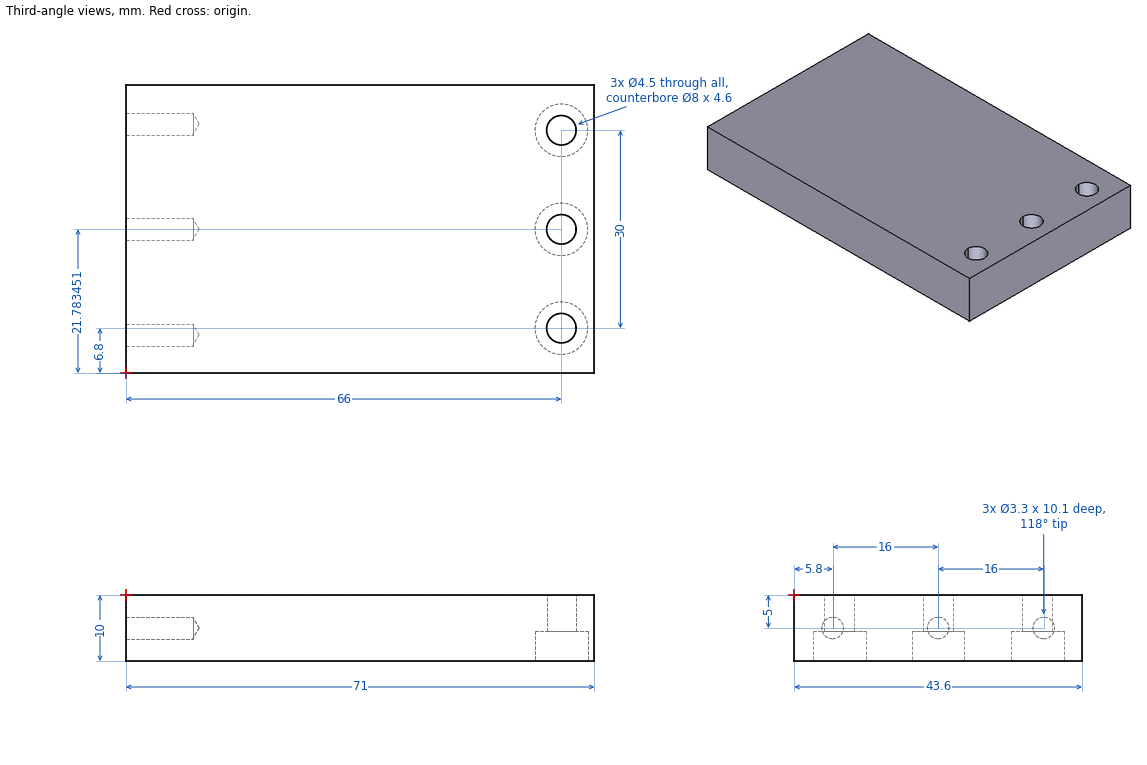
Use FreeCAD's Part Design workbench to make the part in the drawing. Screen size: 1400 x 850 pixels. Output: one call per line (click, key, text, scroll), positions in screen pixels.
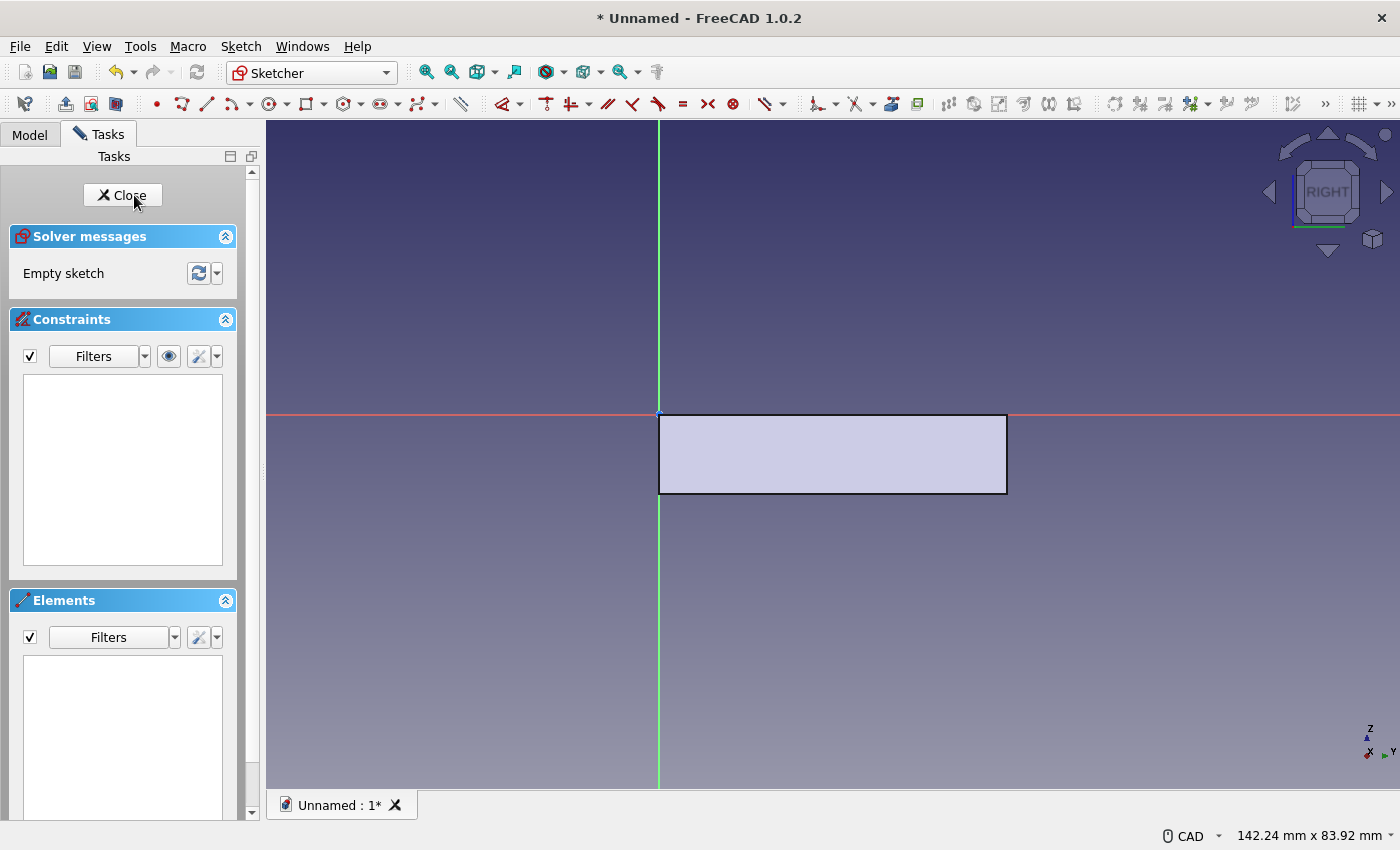
key(q)
key(s)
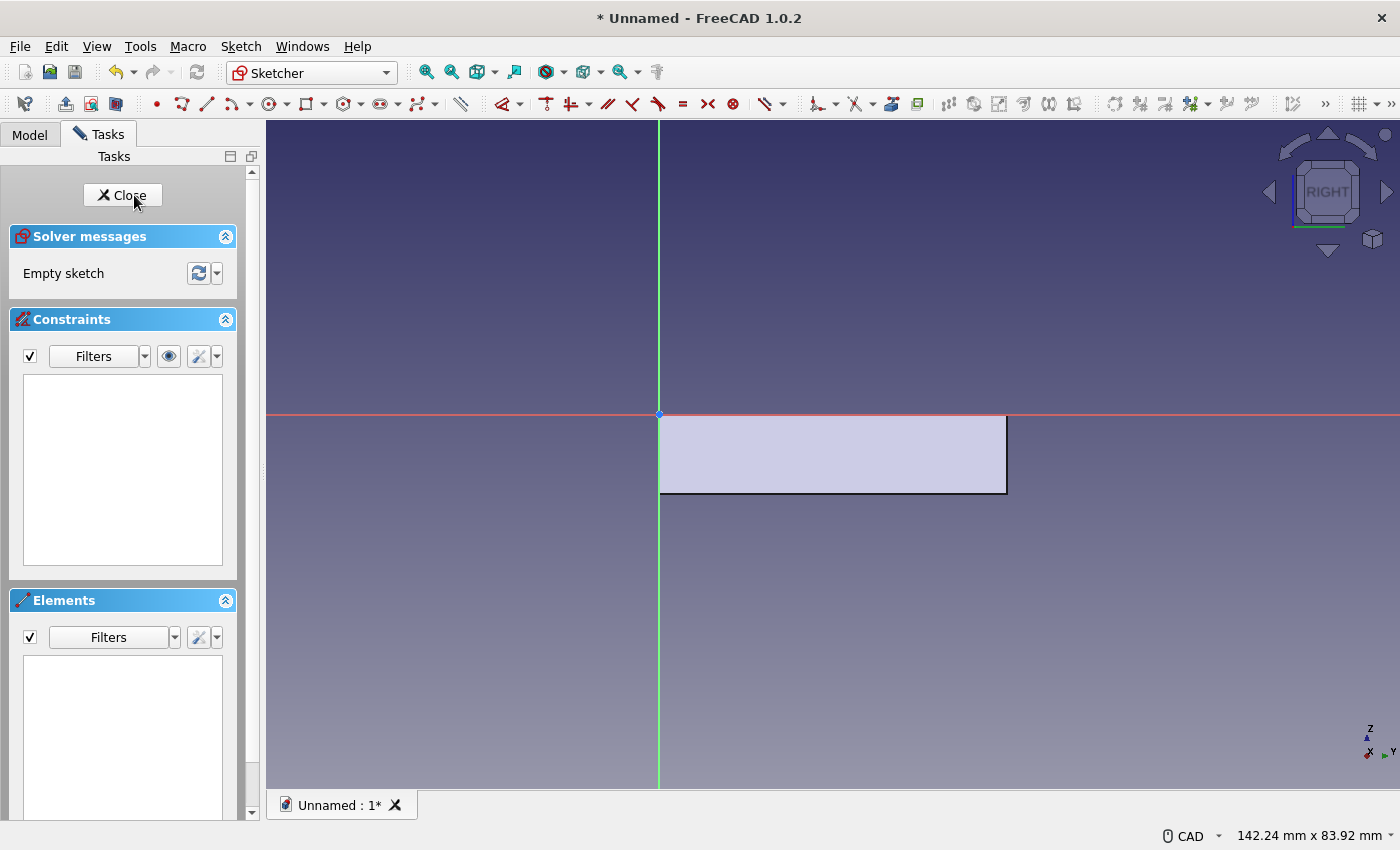
scroll(859, 430, up, 4)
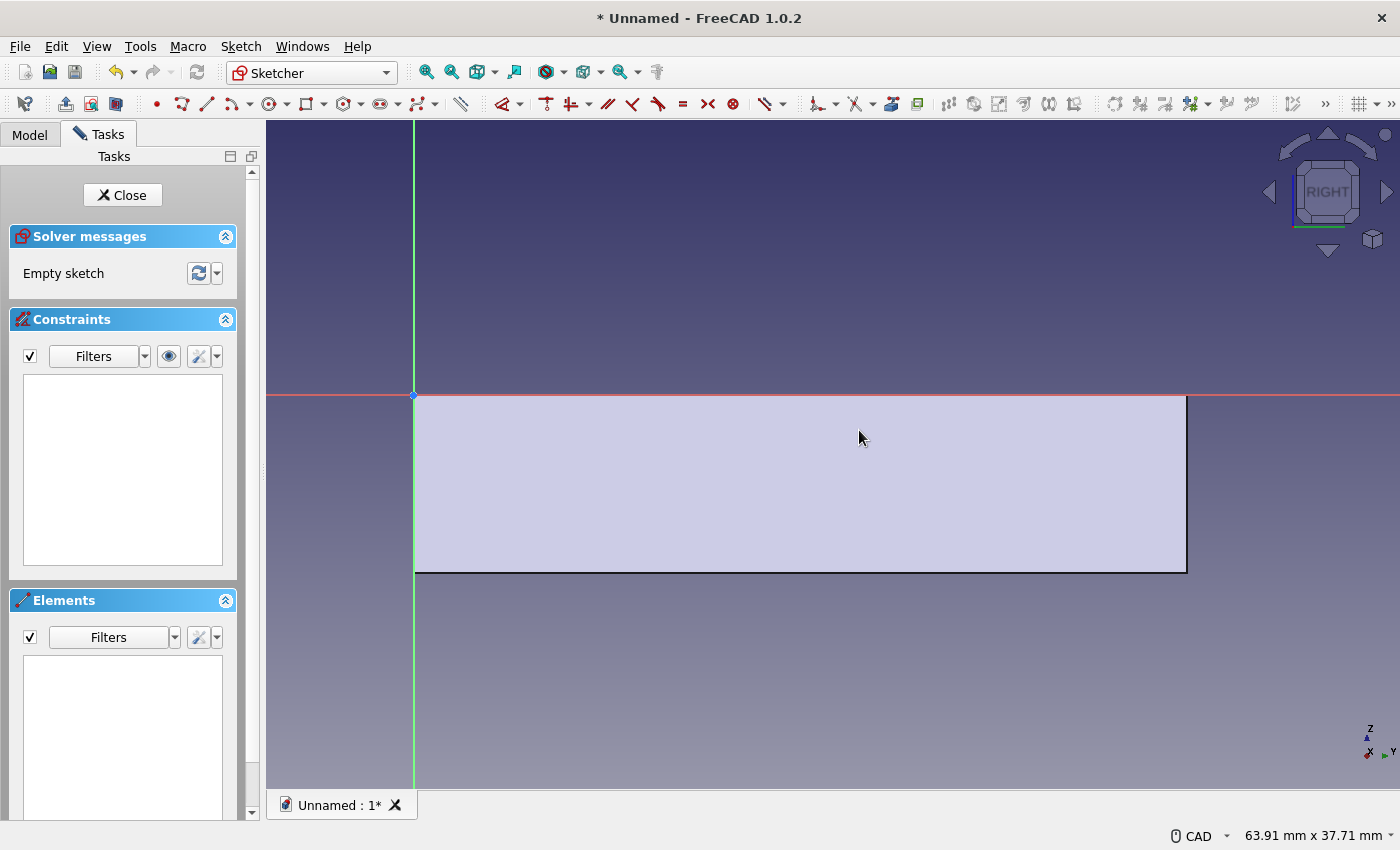
key(g)
key(c)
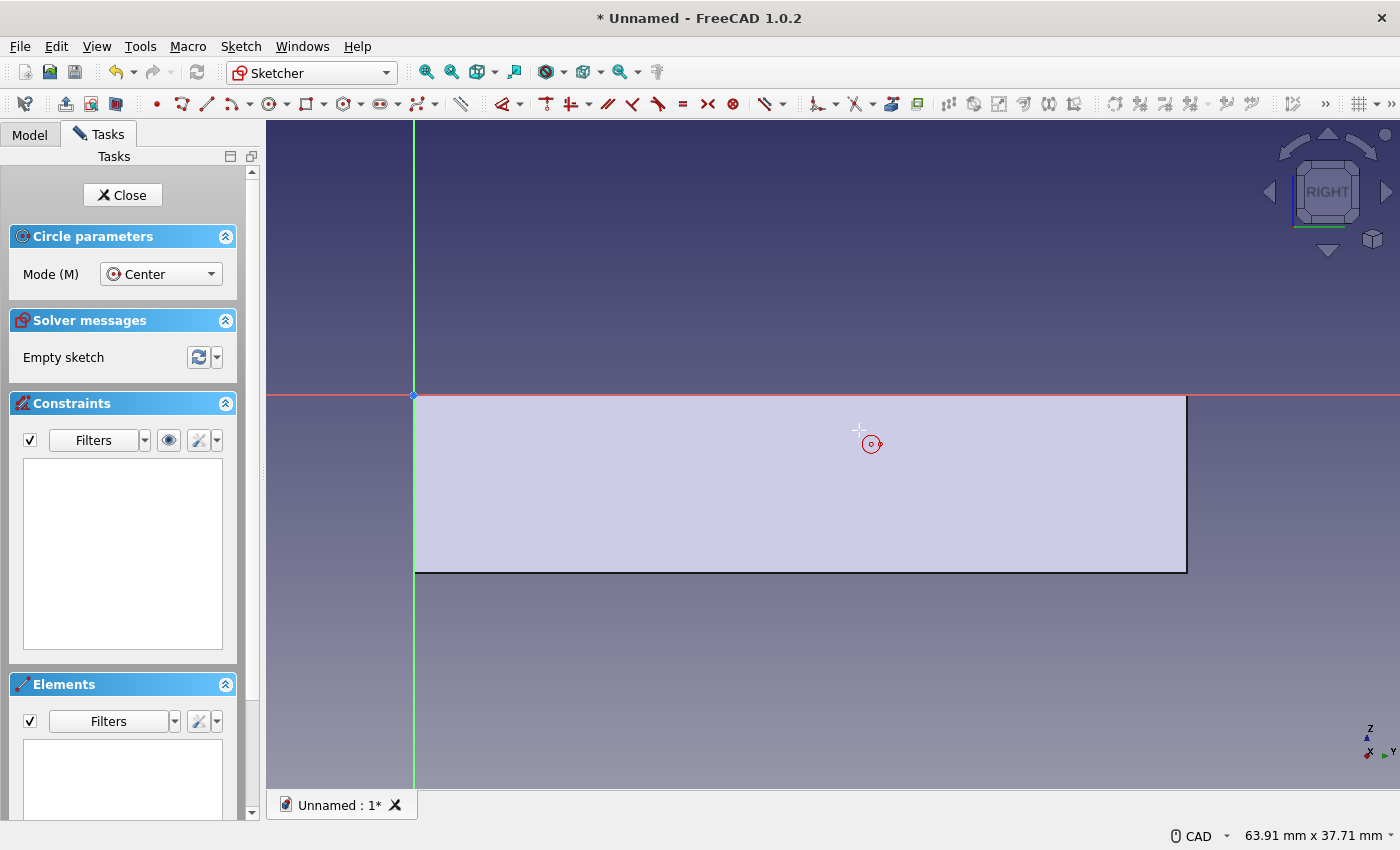
click(1084, 484)
click(1105, 463)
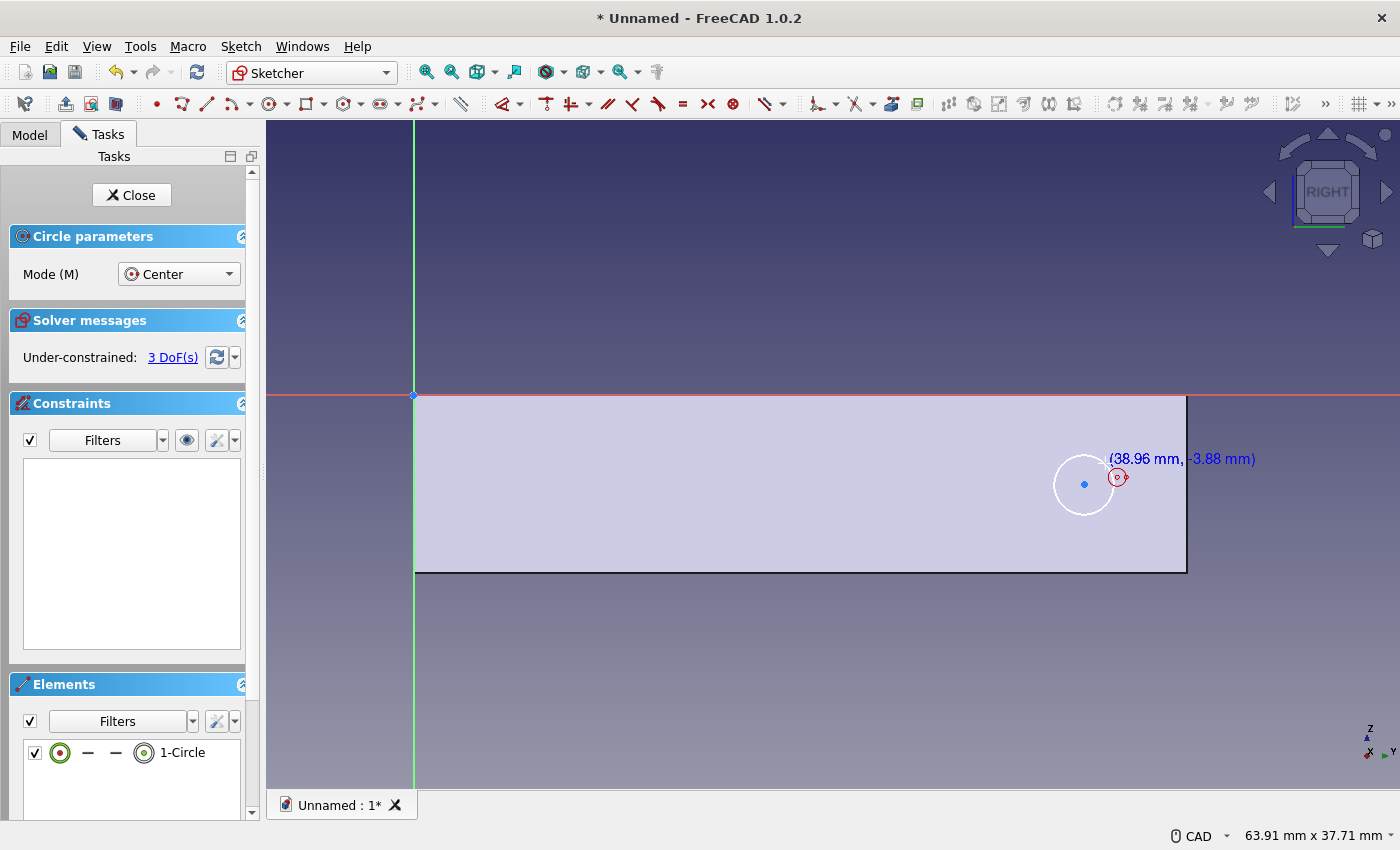
click(800, 484)
click(821, 463)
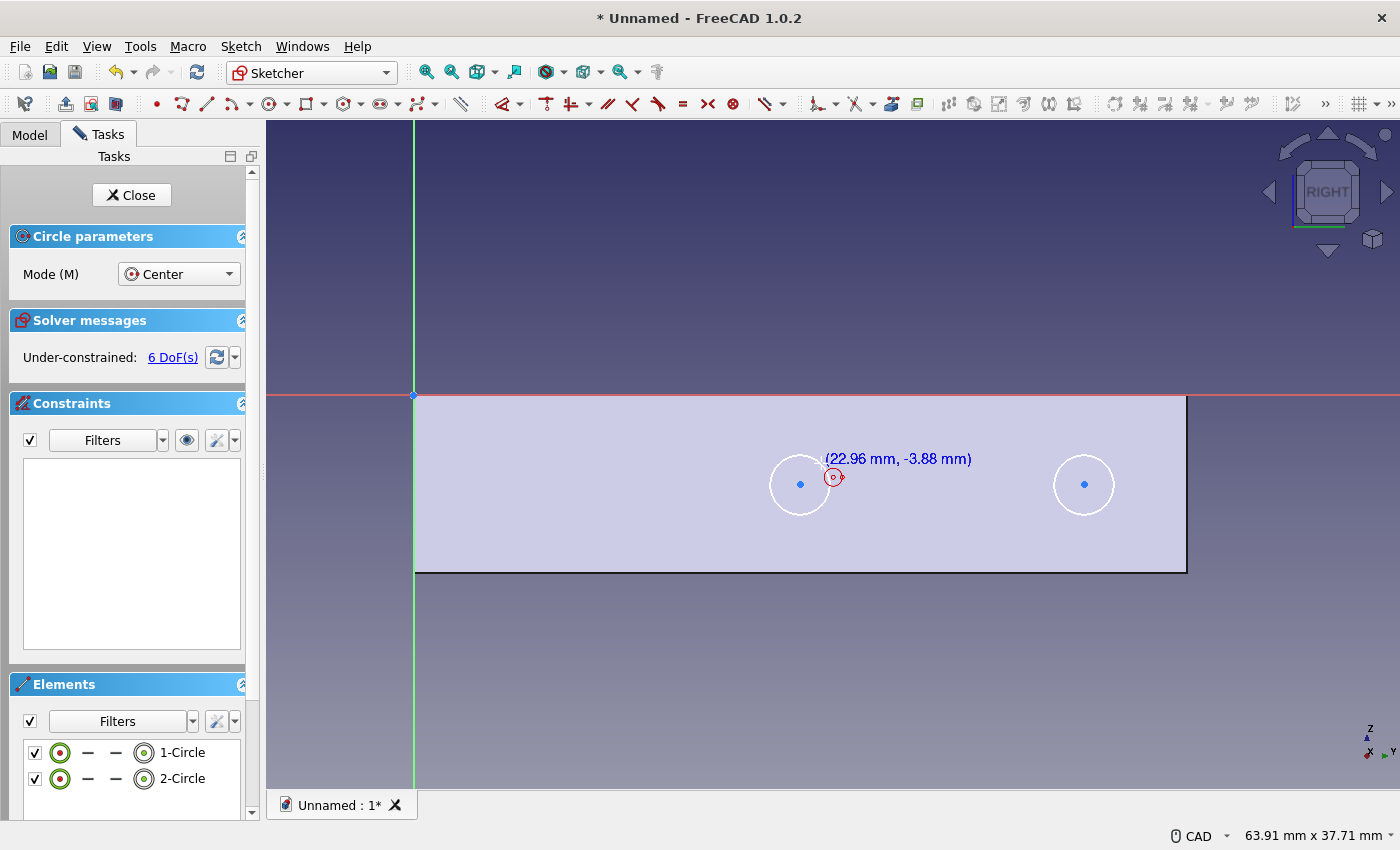
click(517, 484)
click(537, 463)
key(Escape)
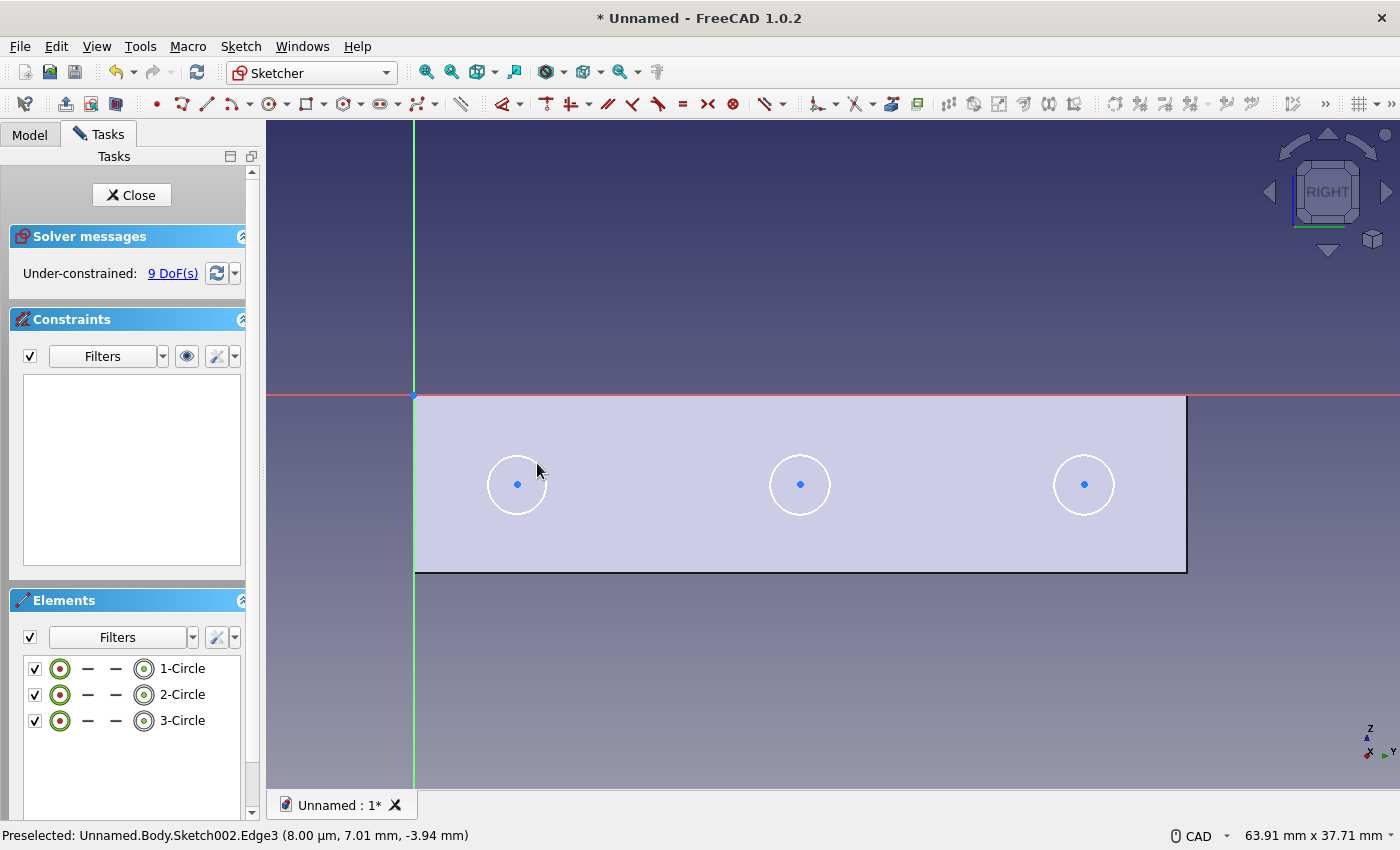
click(1105, 464)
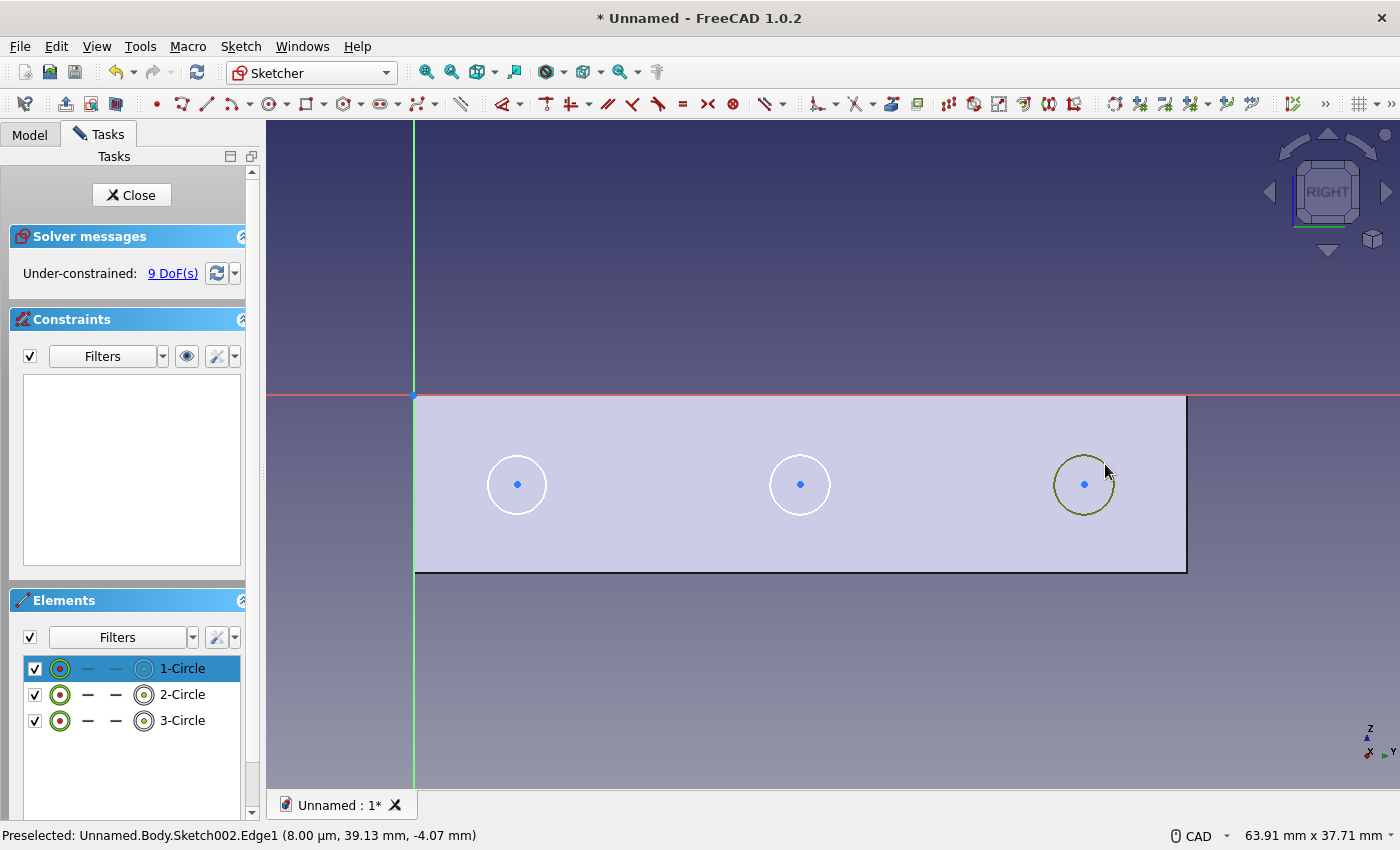
click(821, 464)